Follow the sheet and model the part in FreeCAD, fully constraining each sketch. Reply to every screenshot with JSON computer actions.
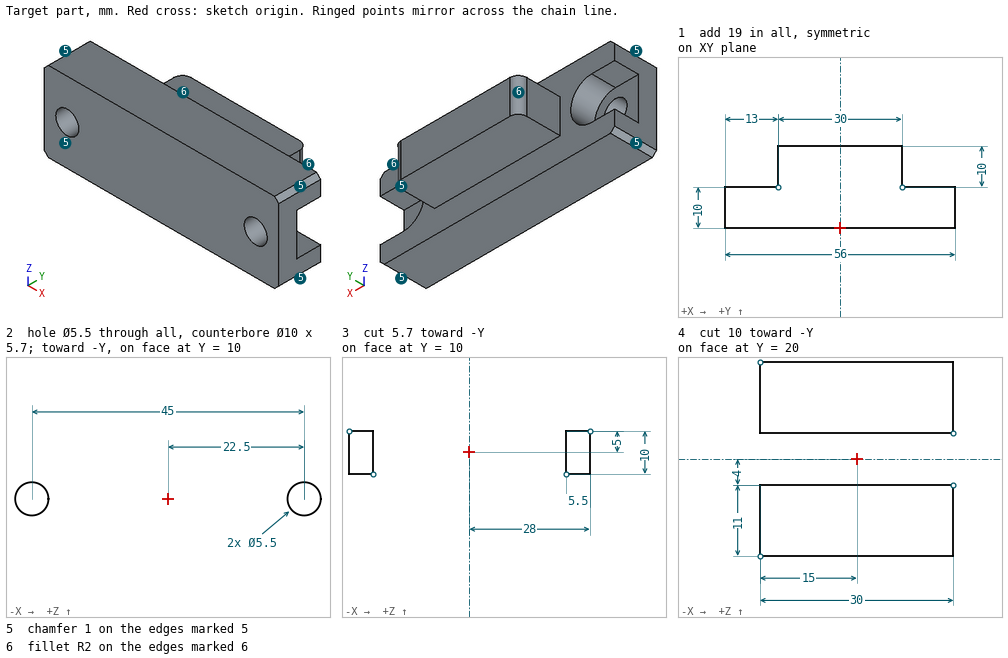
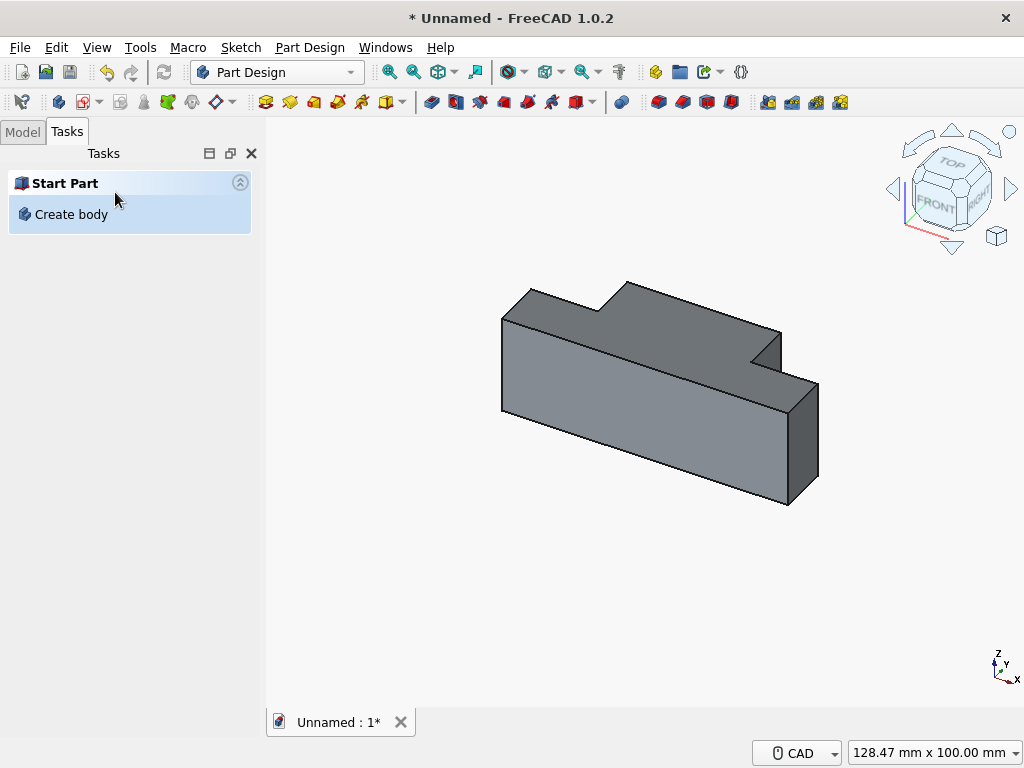
{"action": "key", "text": "4"}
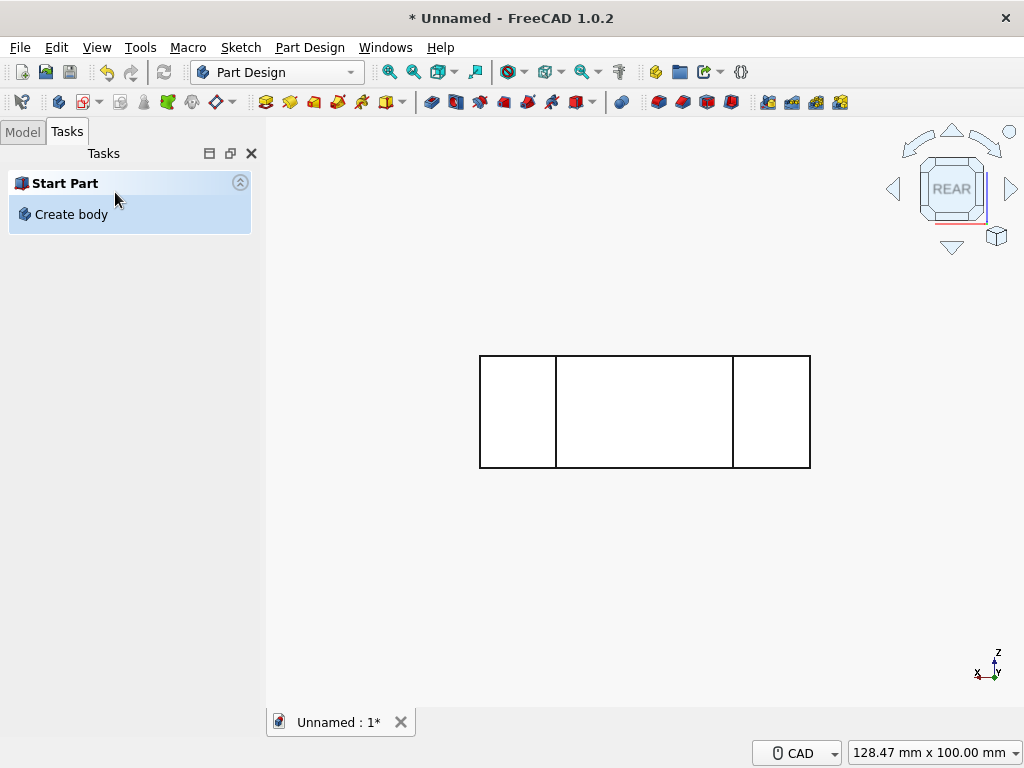
{"action": "left_click", "coordinate": [390, 72]}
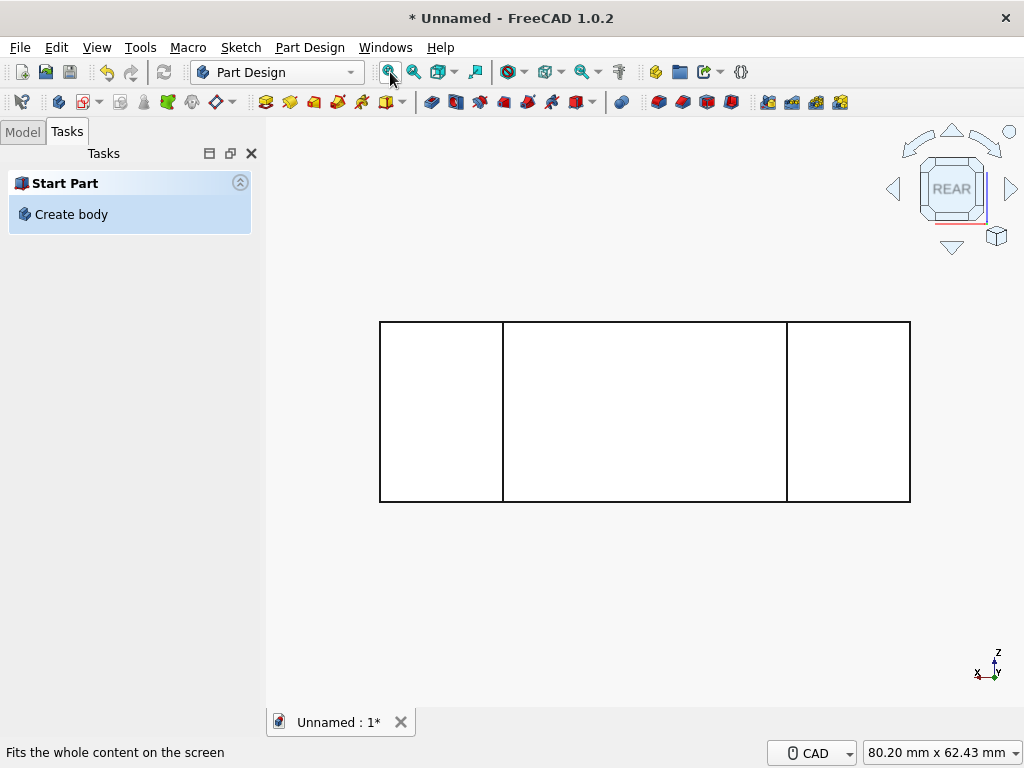
{"action": "left_click", "coordinate": [442, 385]}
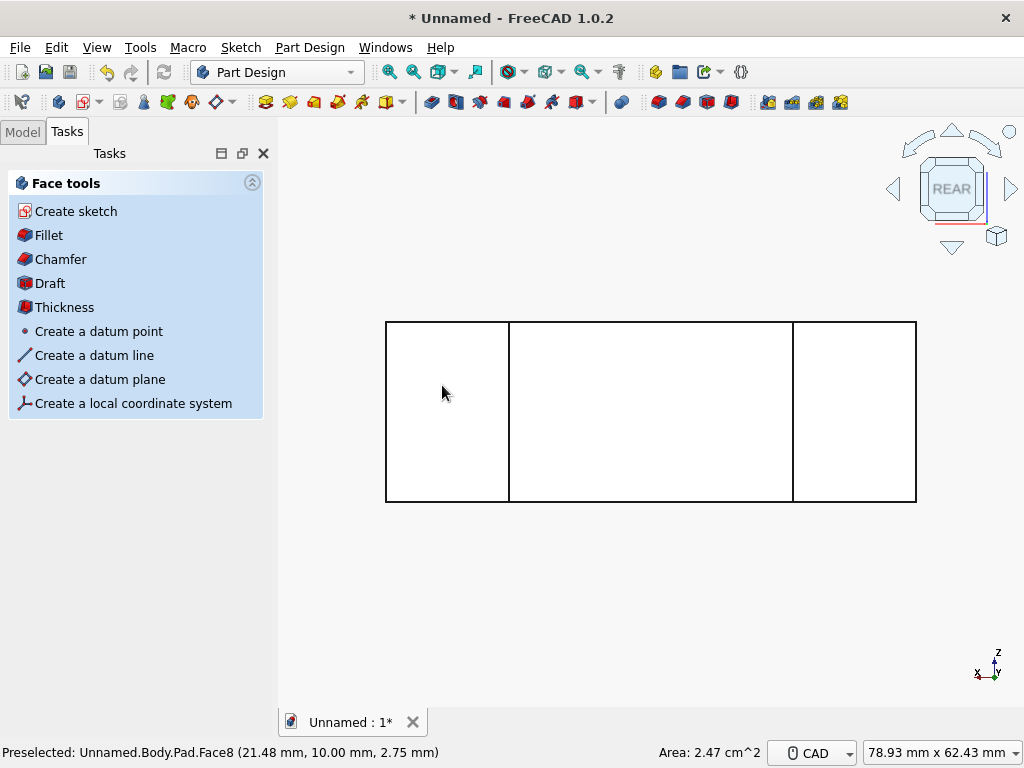
{"action": "left_click", "coordinate": [84, 102]}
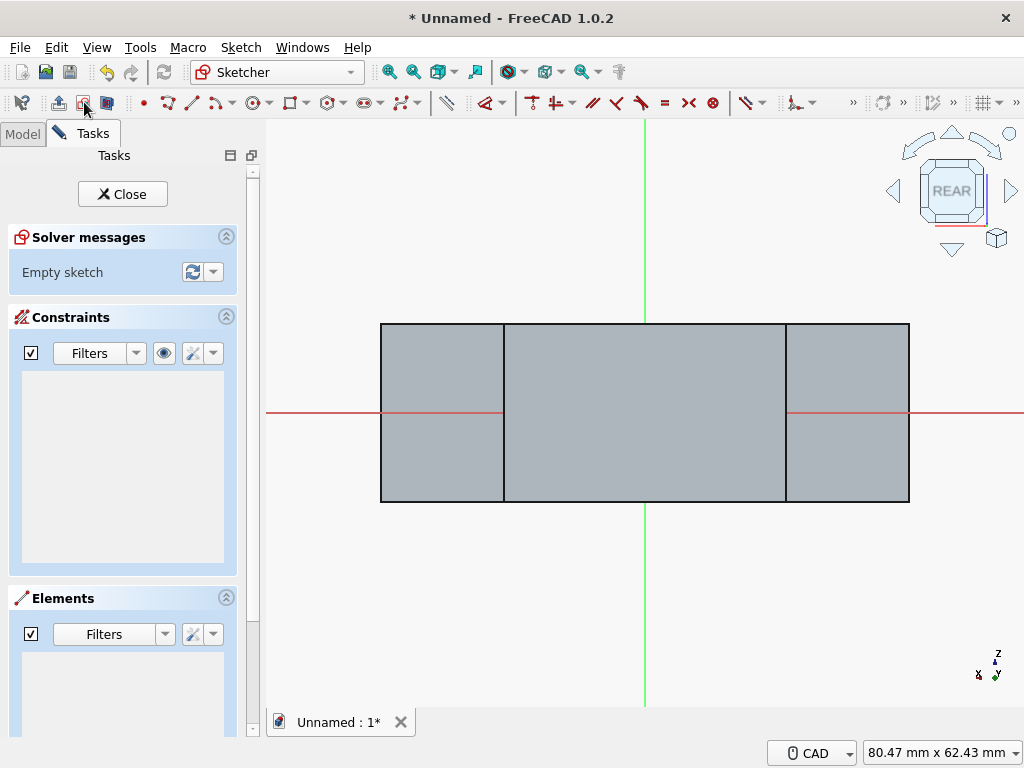
{"action": "scroll", "coordinate": [294, 413], "scroll_direction": "down", "scroll_amount": 1}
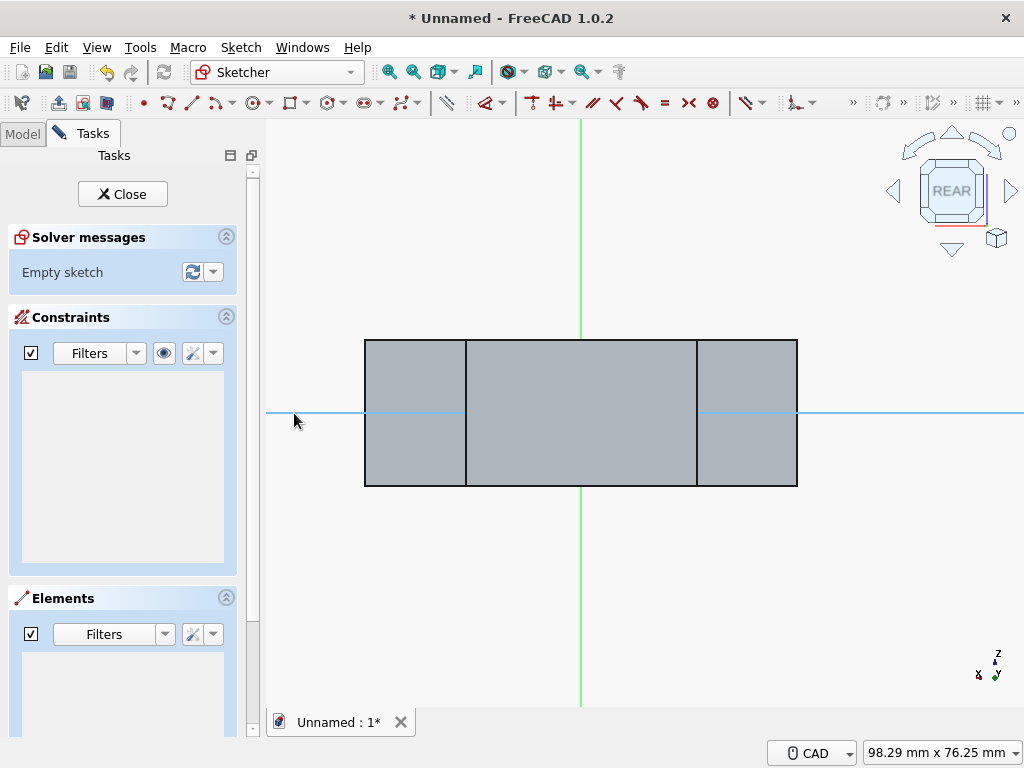
{"action": "left_click", "coordinate": [254, 104]}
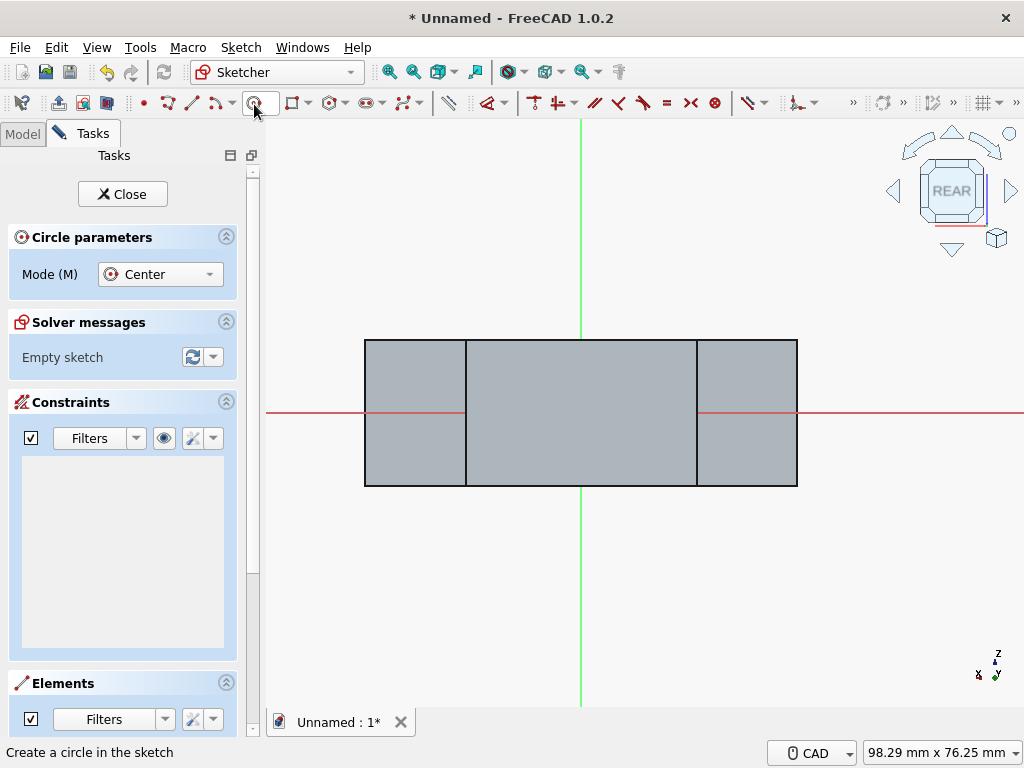
{"action": "left_click", "coordinate": [755, 413]}
{"action": "left_click", "coordinate": [770, 398]}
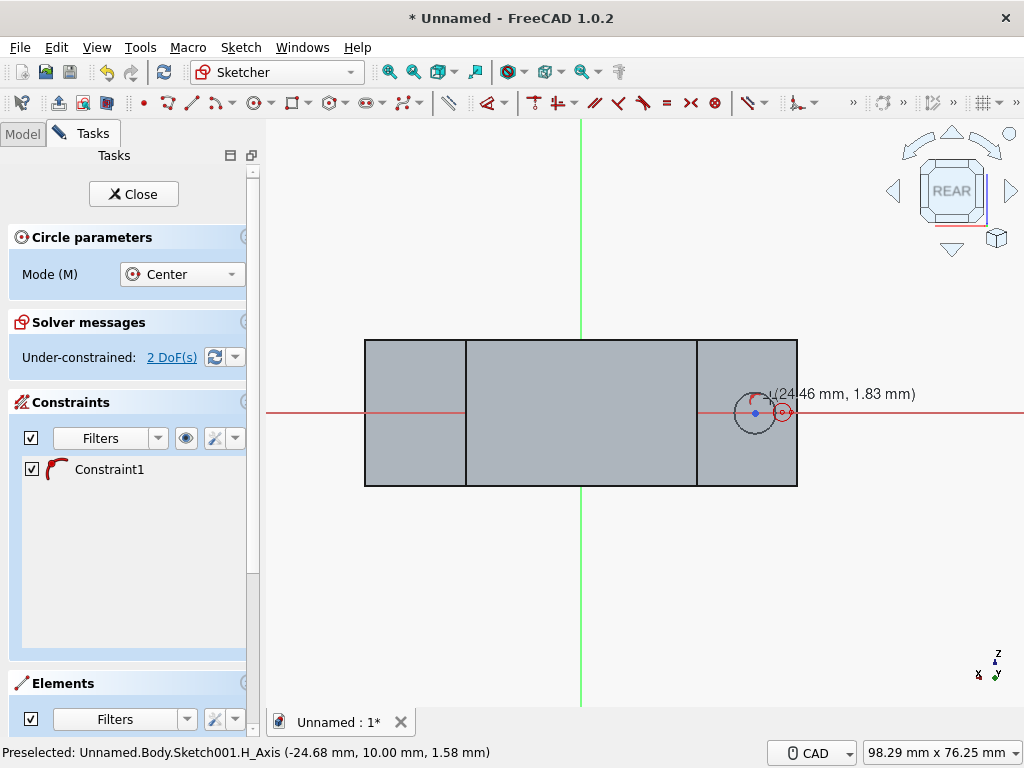
{"action": "left_click", "coordinate": [408, 413]}
{"action": "left_click", "coordinate": [423, 398]}
{"action": "key", "text": "Escape"}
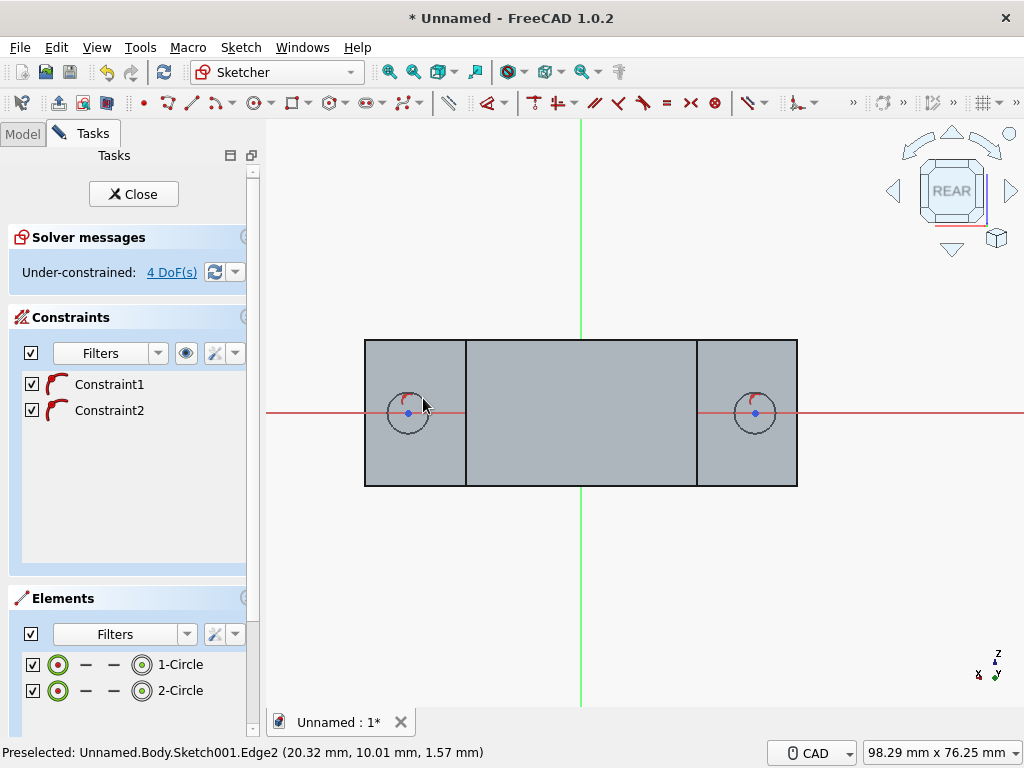
{"action": "left_click", "coordinate": [770, 398]}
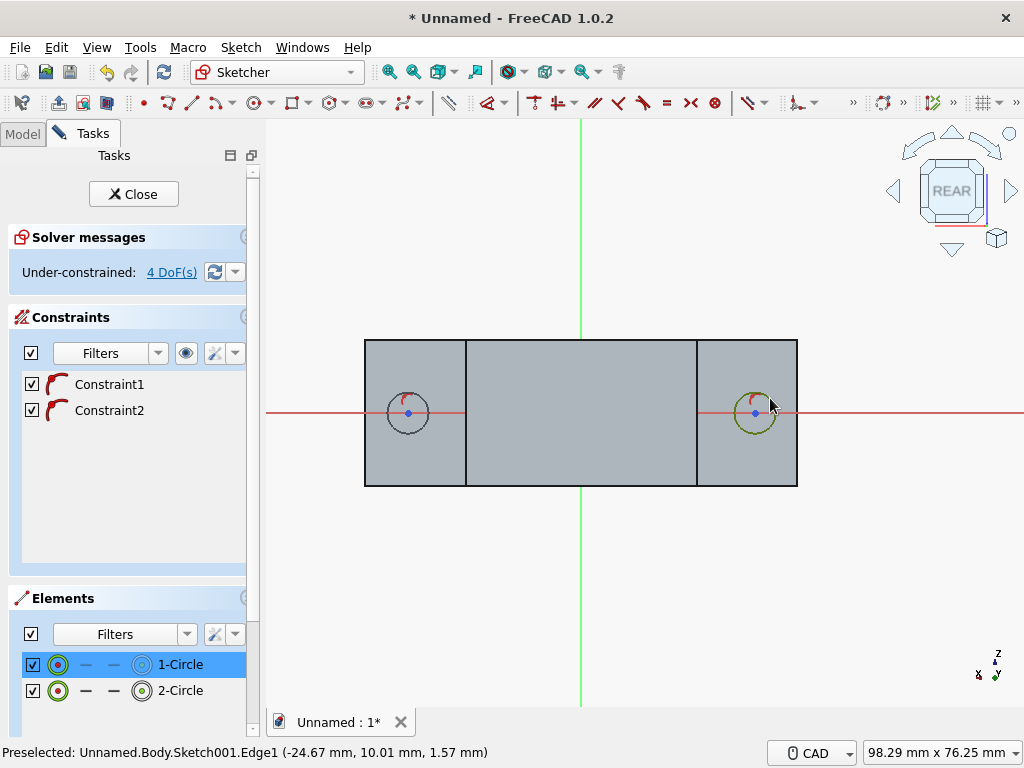
{"action": "left_click", "coordinate": [423, 398]}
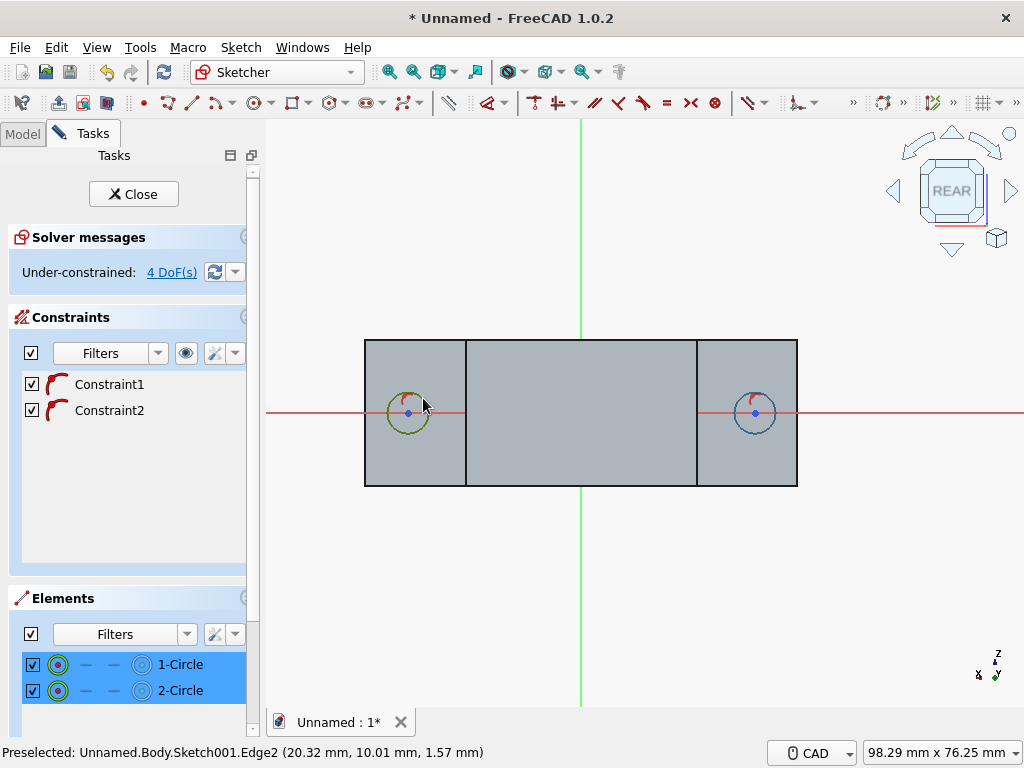
{"action": "left_click", "coordinate": [668, 104]}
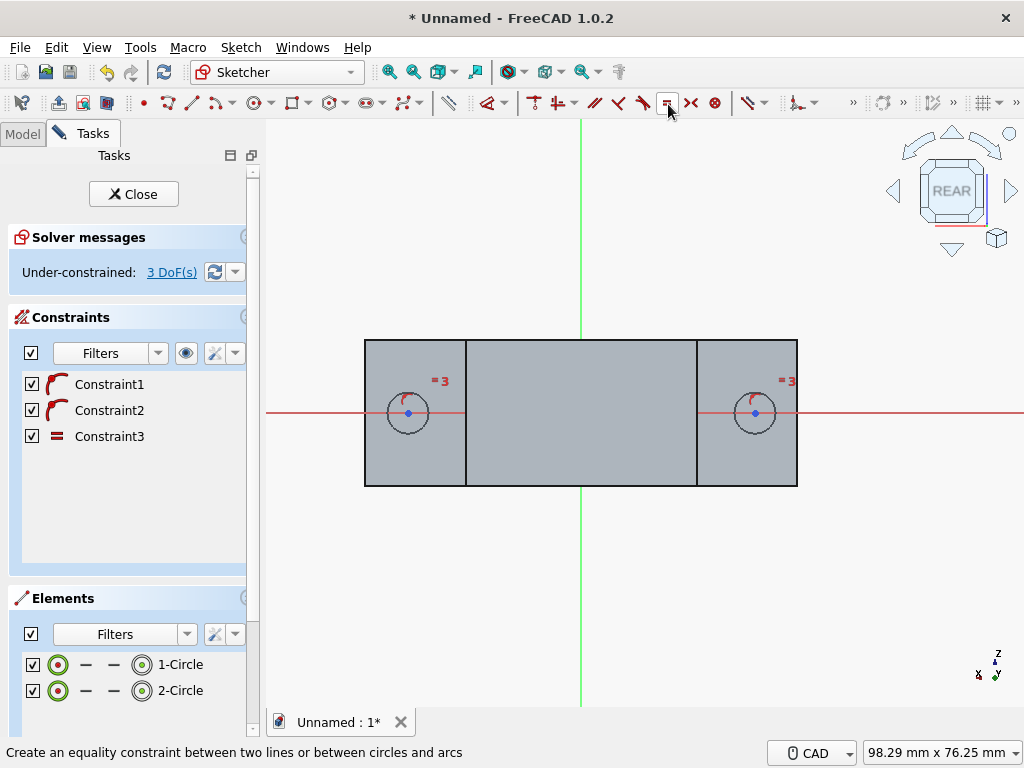
{"action": "left_click", "coordinate": [488, 104]}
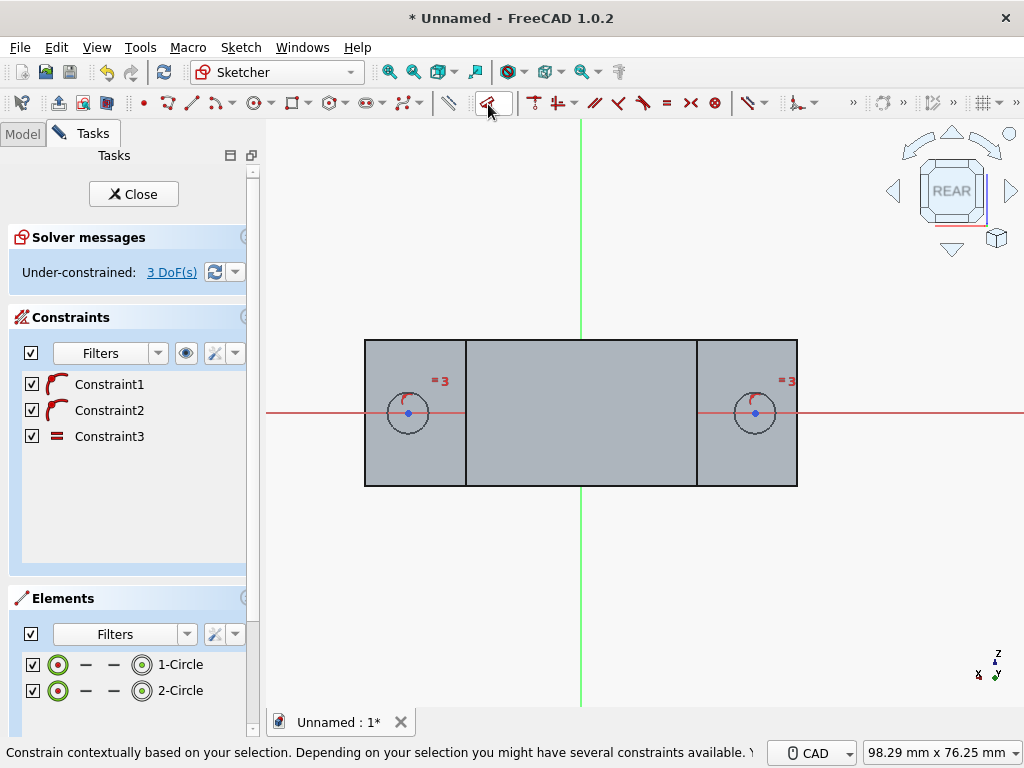
{"action": "left_click", "coordinate": [770, 398]}
{"action": "left_click", "coordinate": [793, 375]}